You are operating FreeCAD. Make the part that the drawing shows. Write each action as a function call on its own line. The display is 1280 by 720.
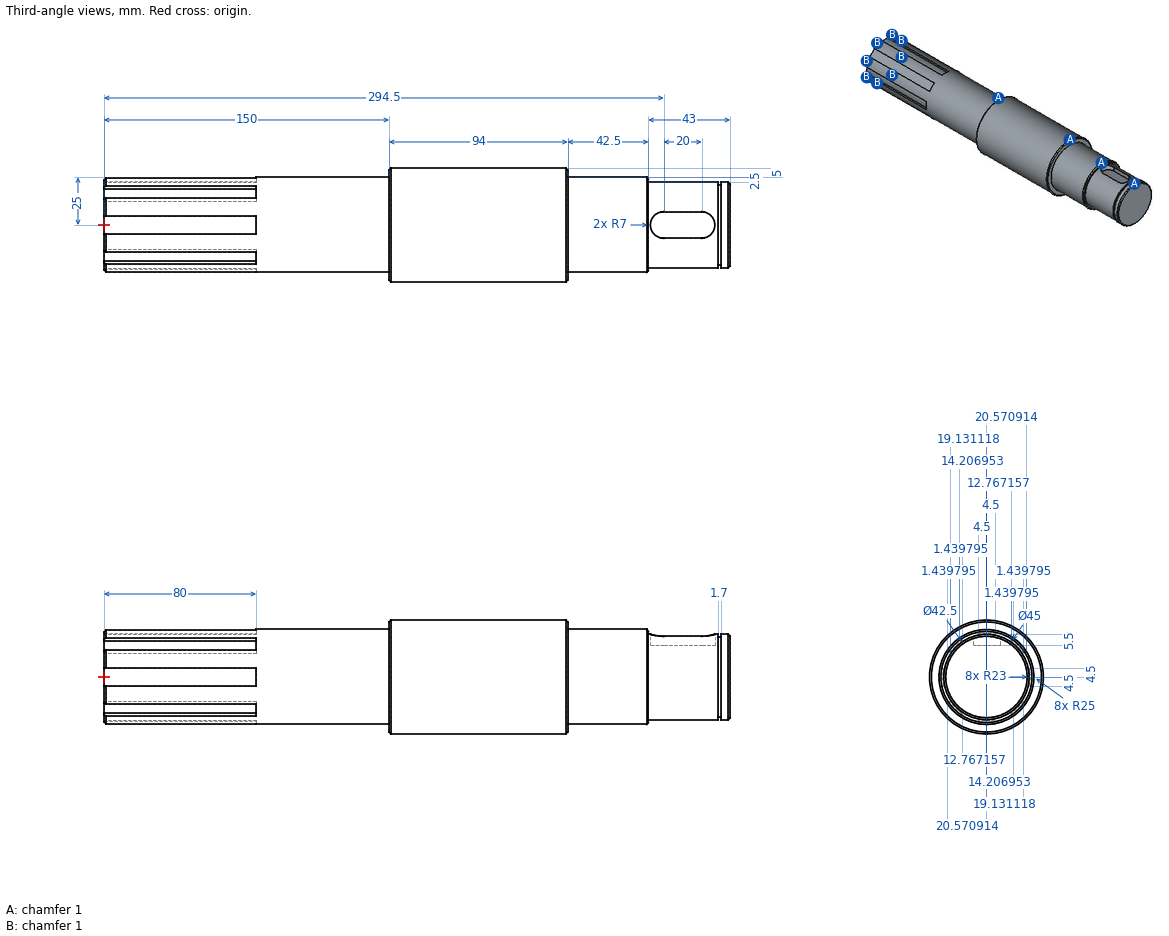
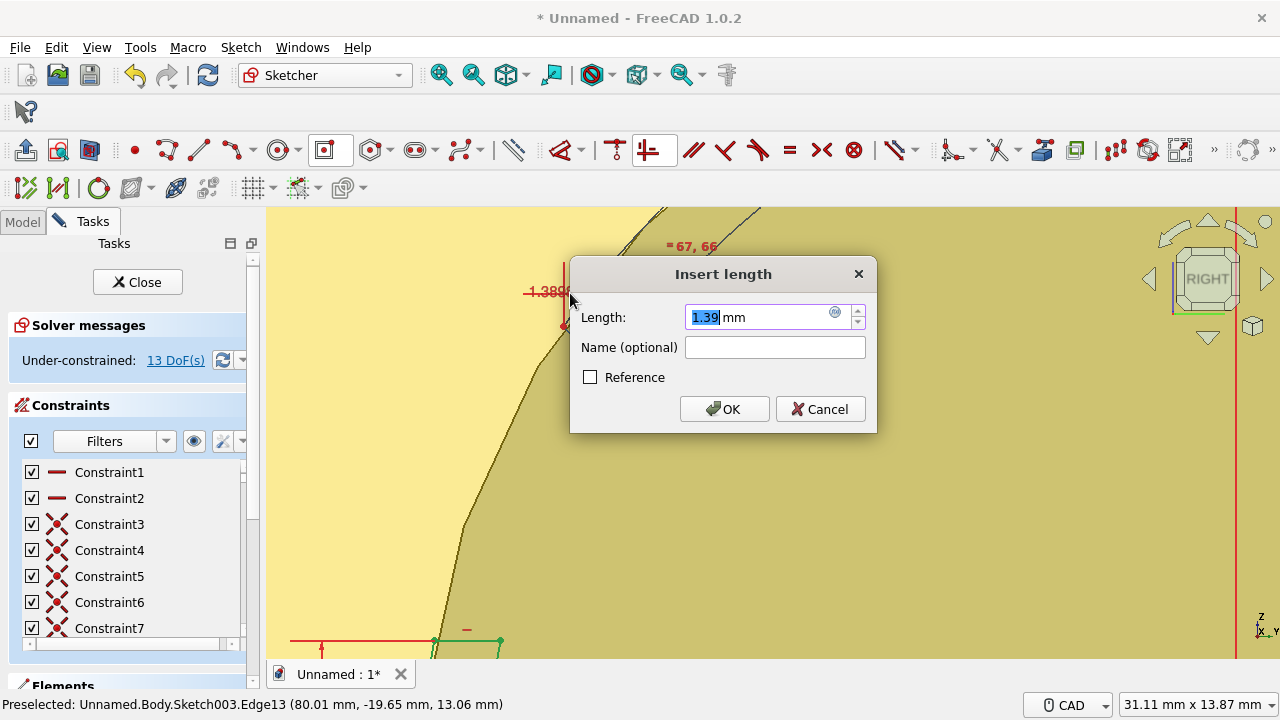
text(1.439795)
key(Return)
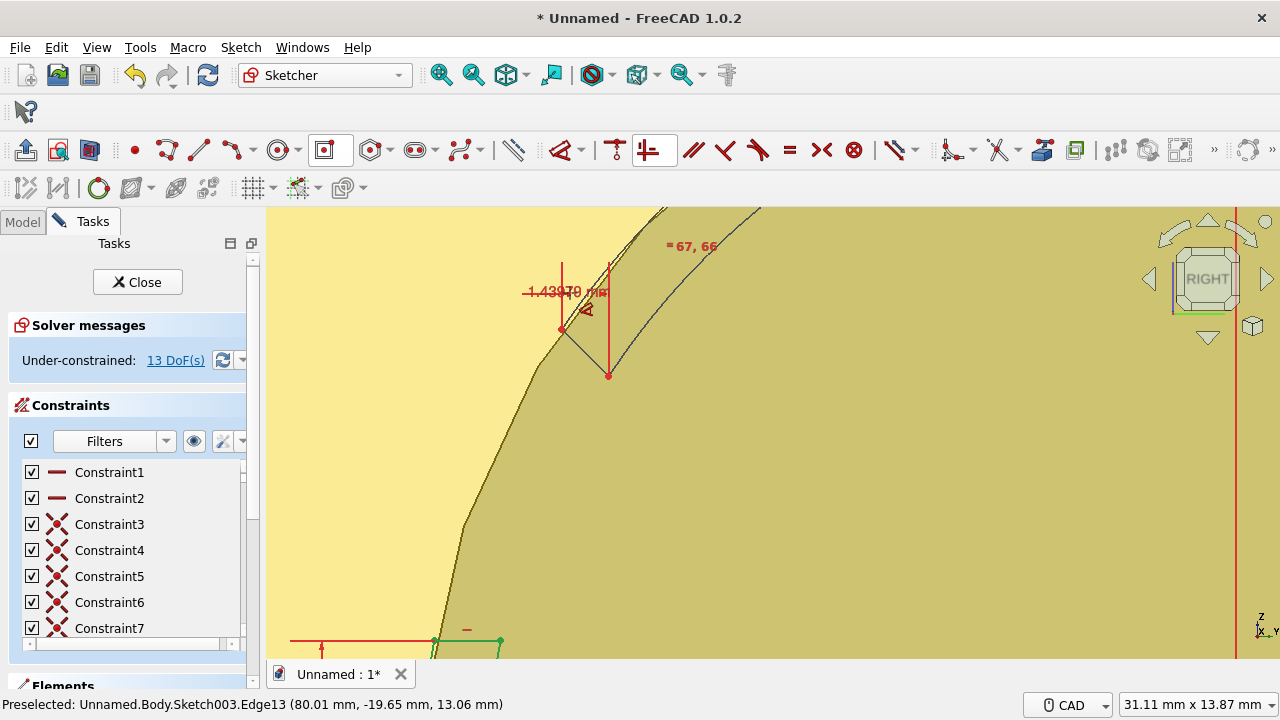
scroll(599, 363, down, 9)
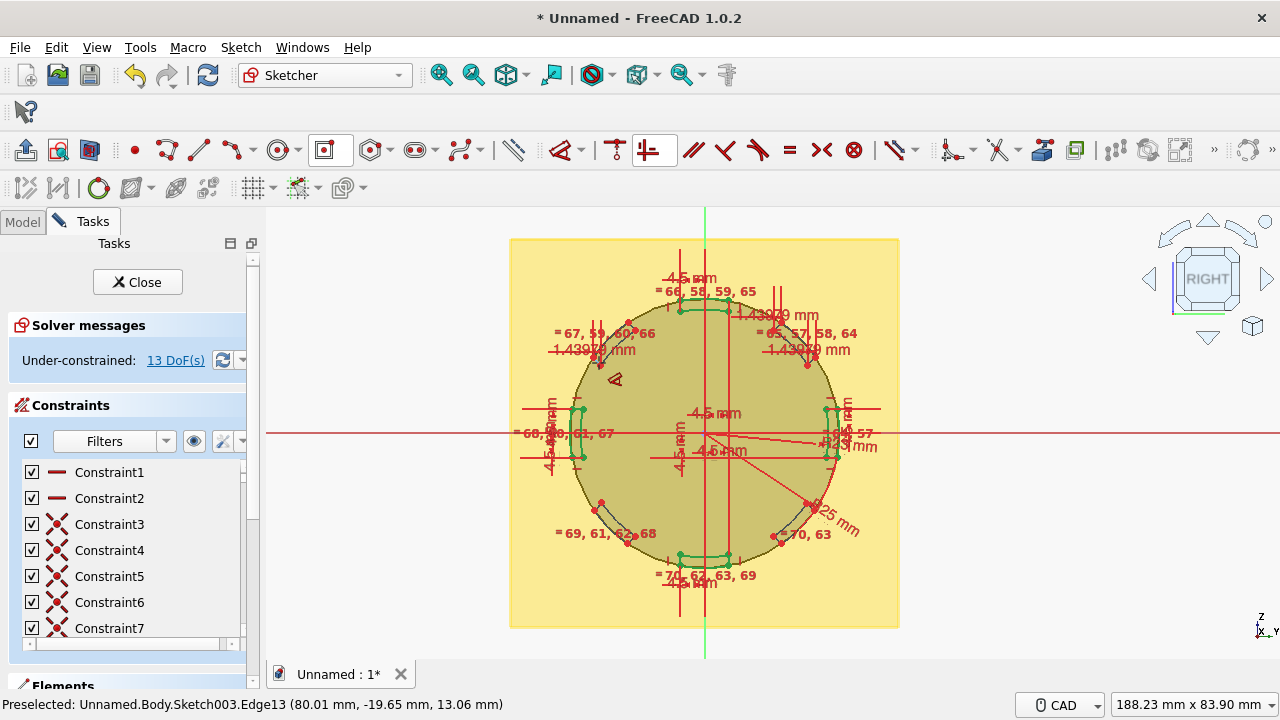
scroll(631, 325, up, 9)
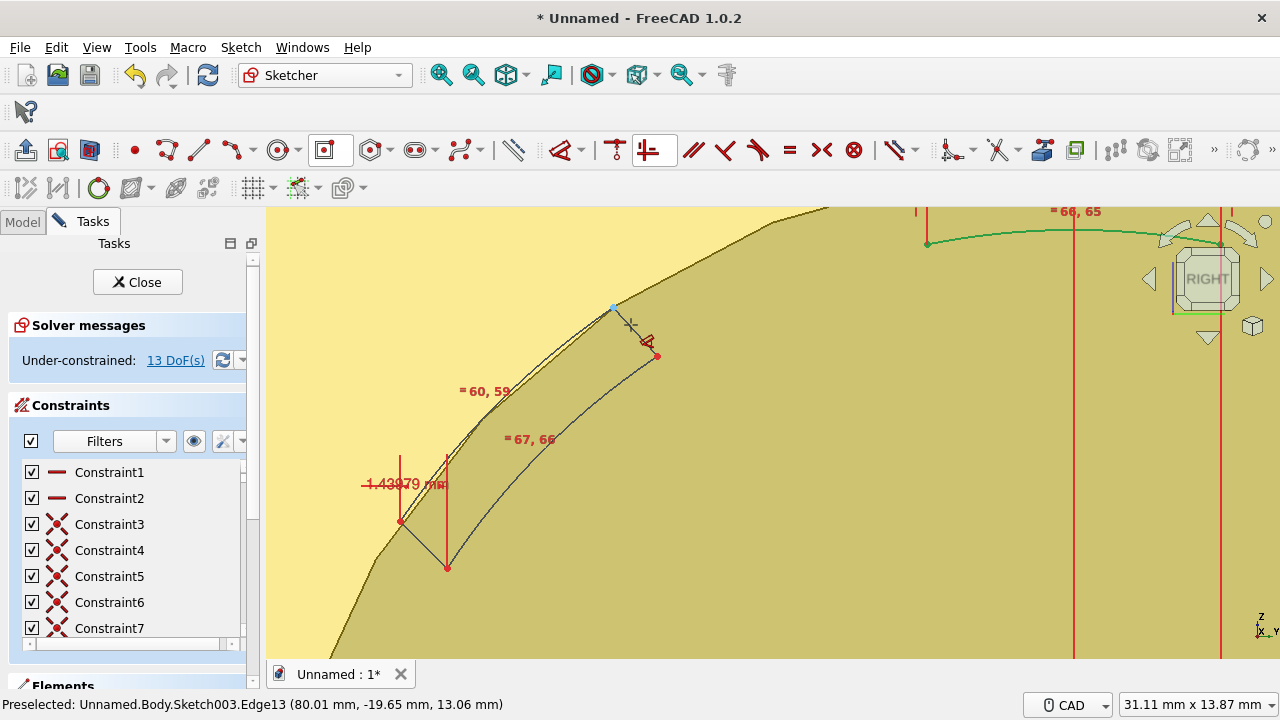
click(627, 322)
click(635, 274)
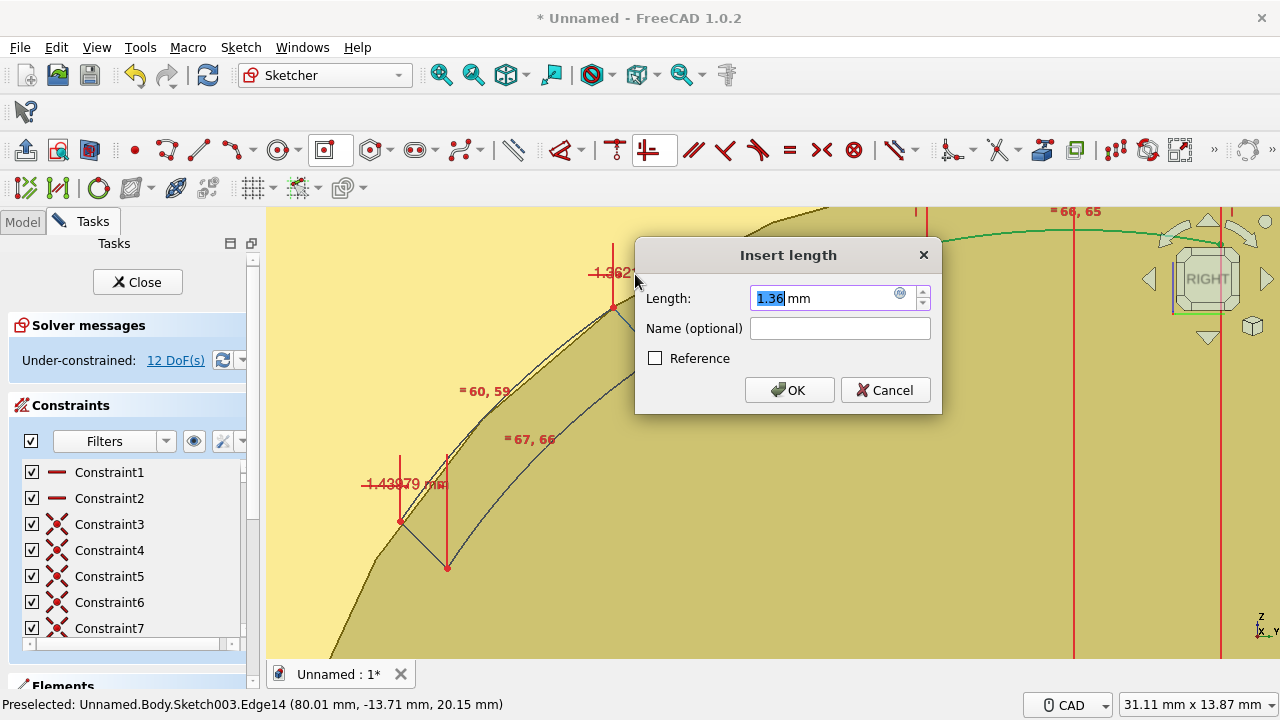
text(1.439795)
key(Return)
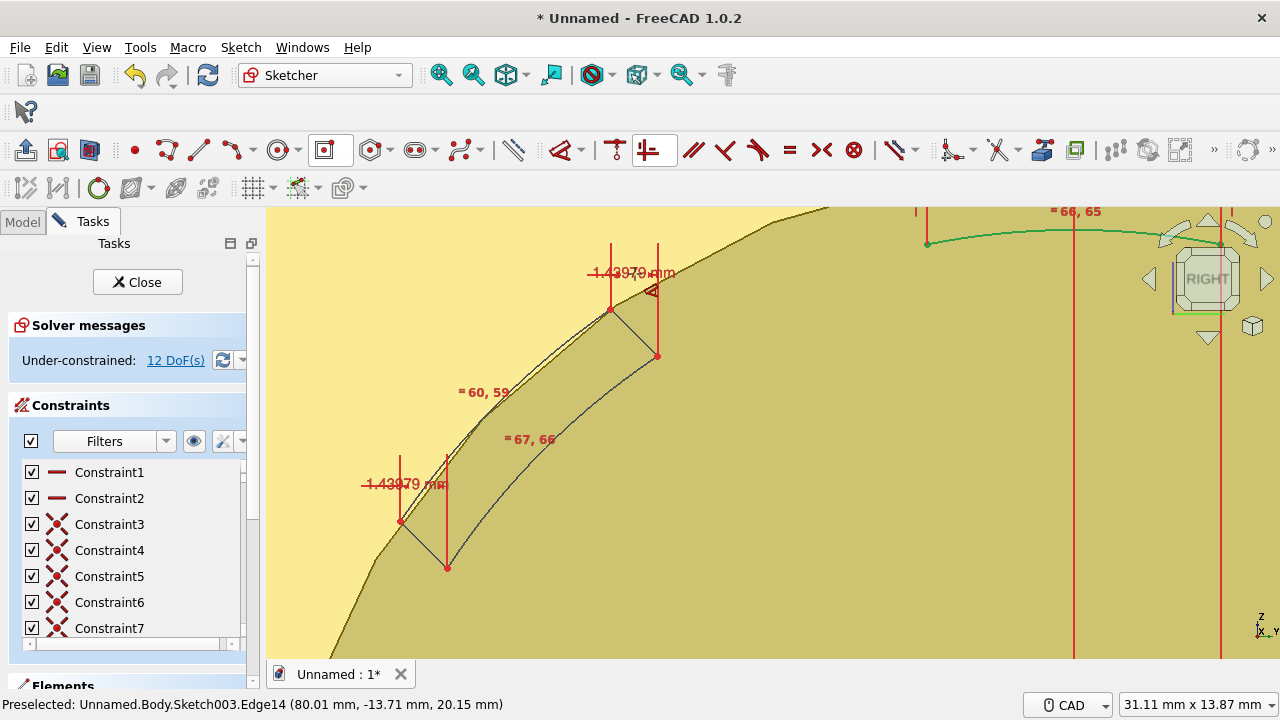
scroll(631, 325, down, 9)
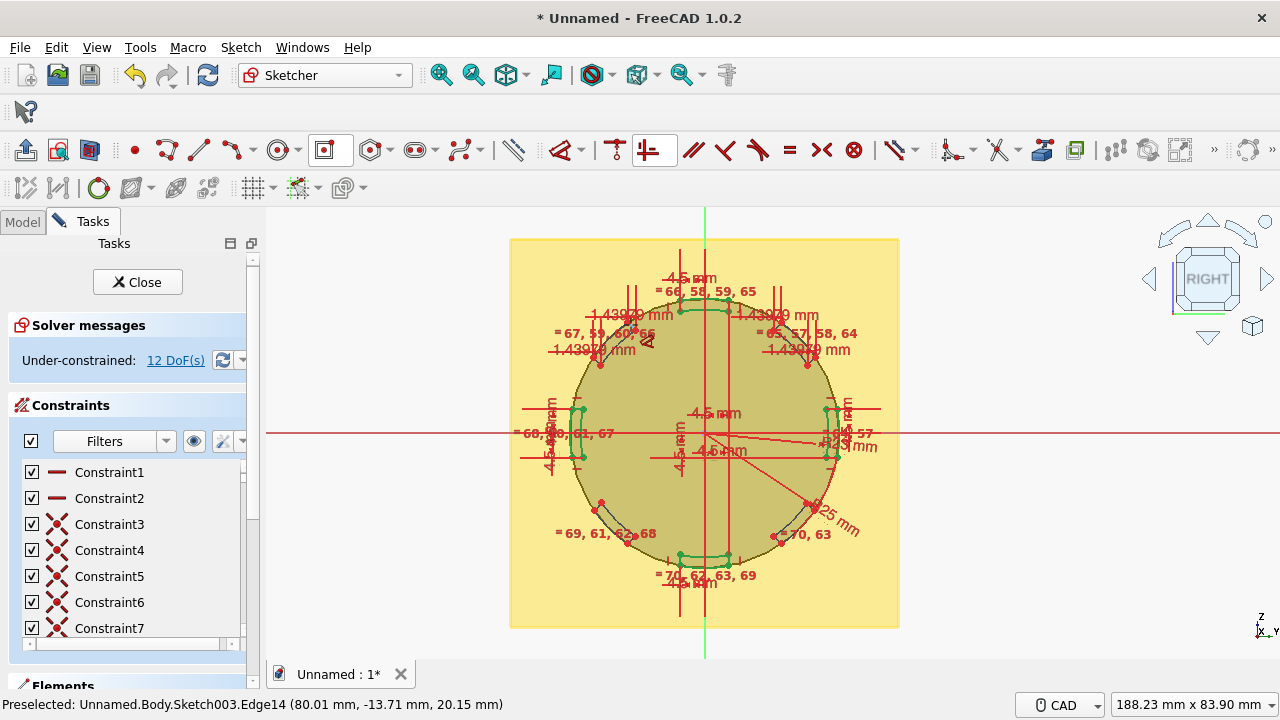
scroll(633, 539, up, 9)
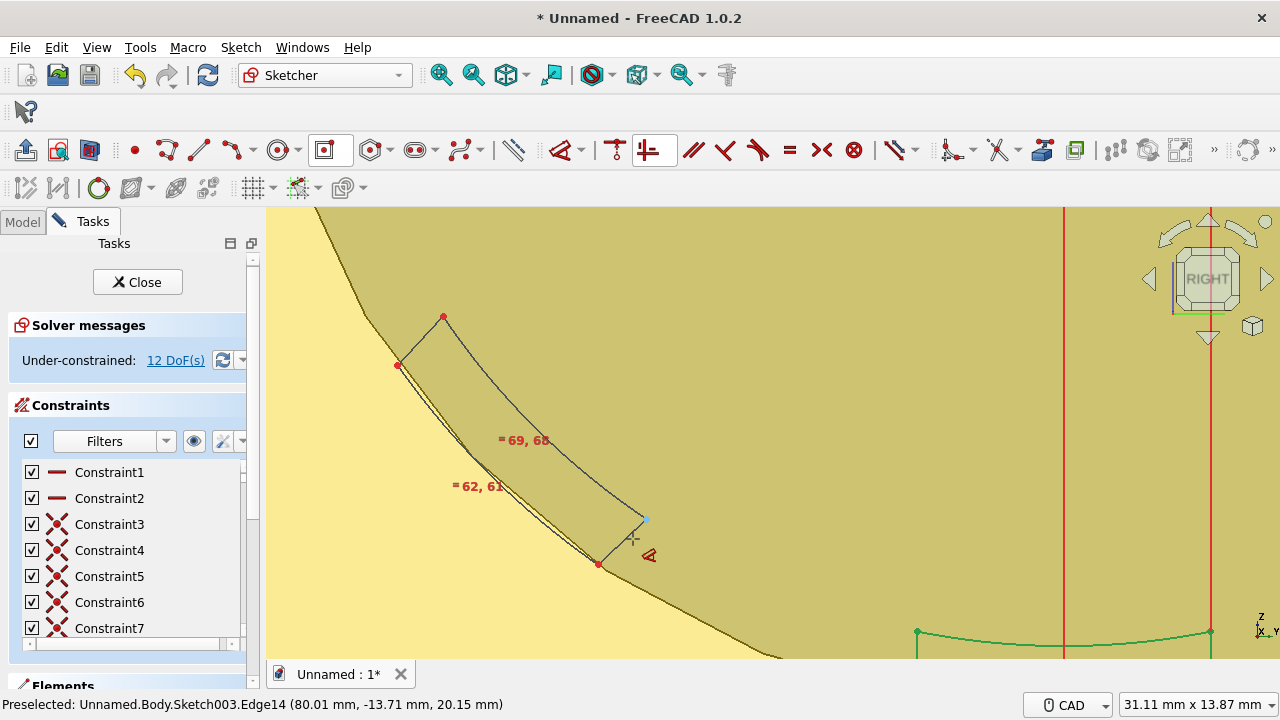
click(632, 533)
click(622, 599)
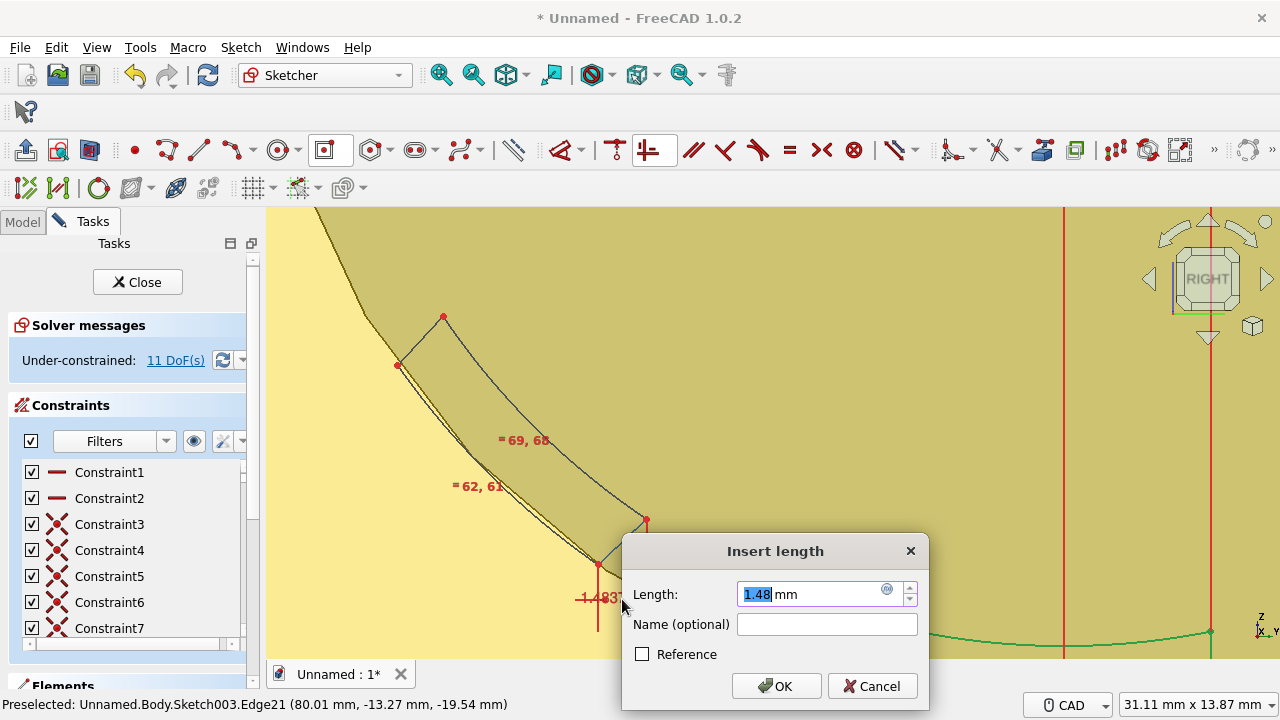
text(1.439795)
key(Return)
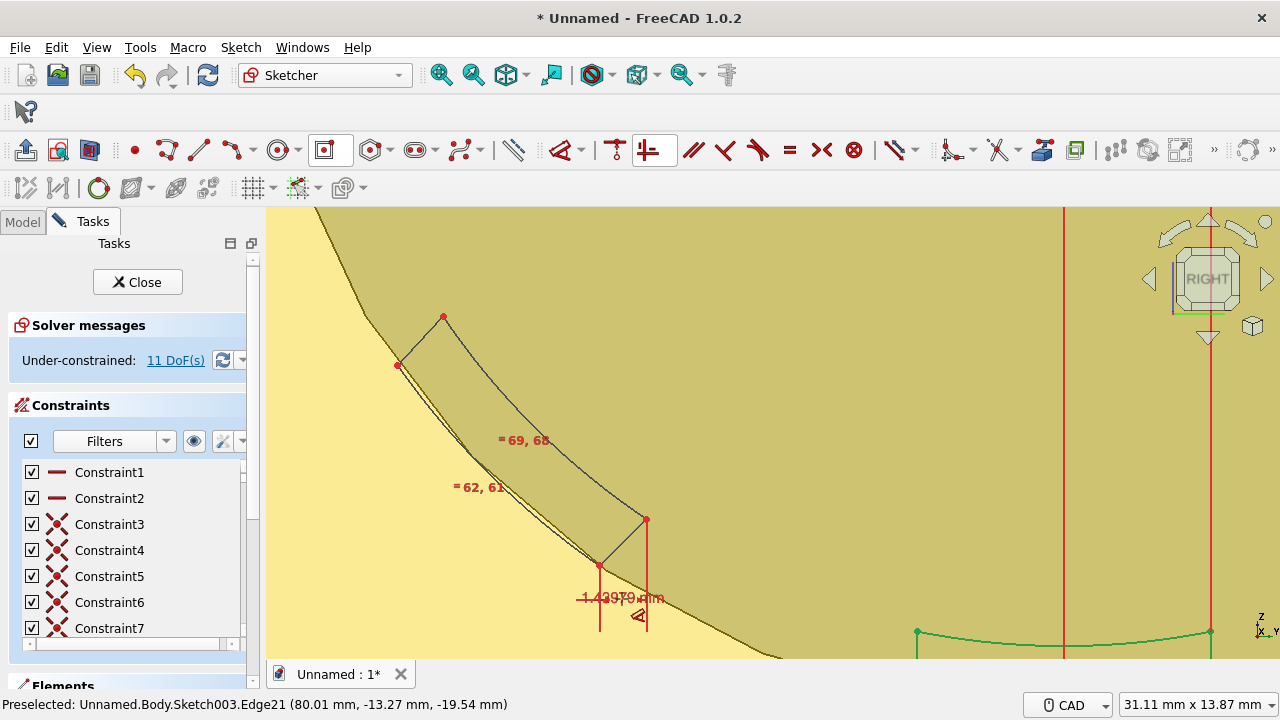
click(411, 351)
click(405, 400)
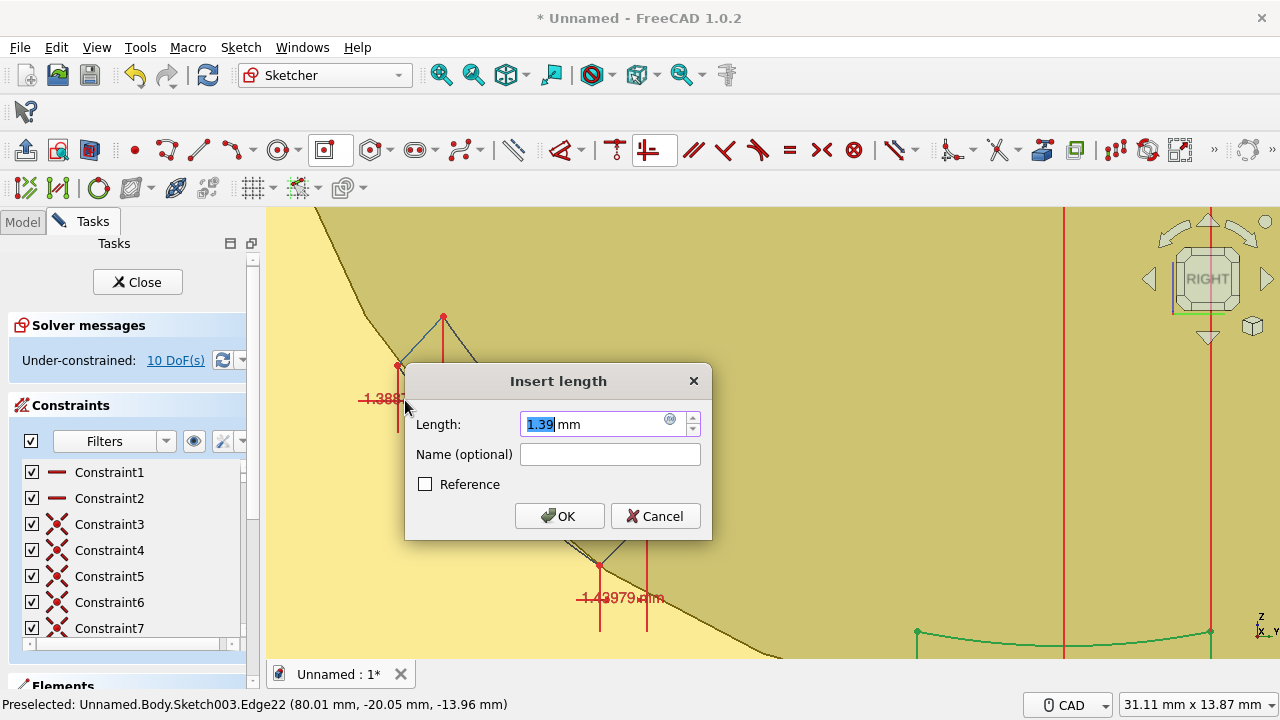
text(1.439795)
key(Return)